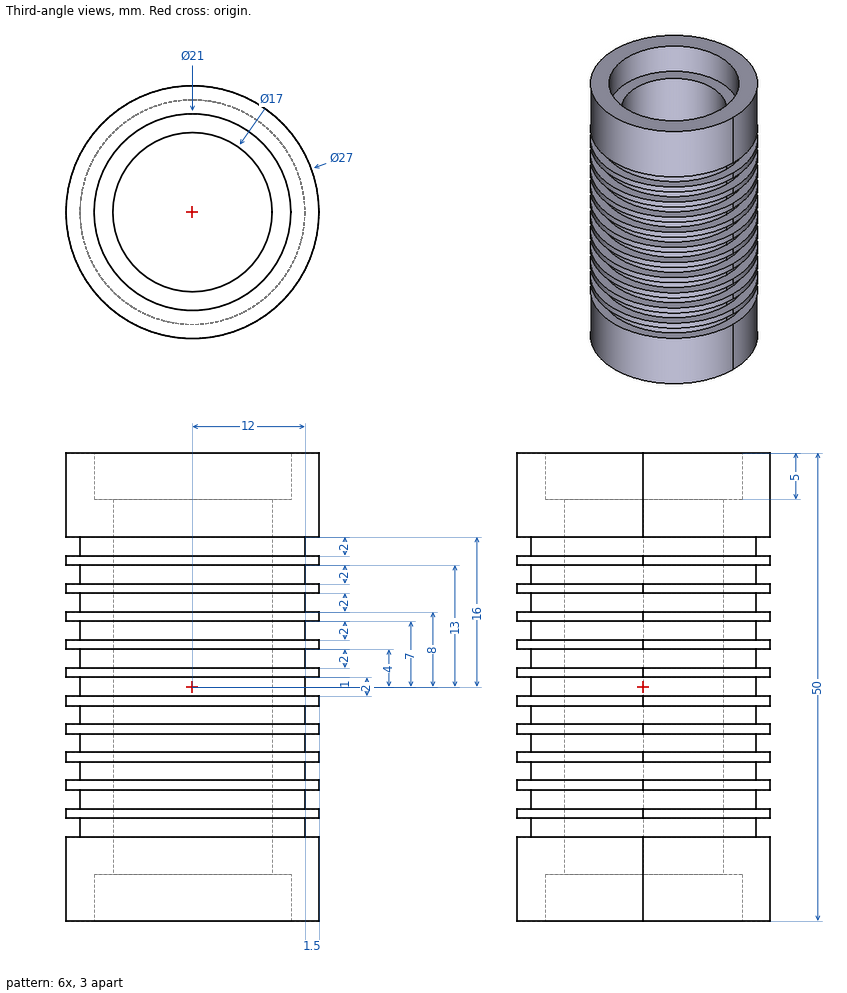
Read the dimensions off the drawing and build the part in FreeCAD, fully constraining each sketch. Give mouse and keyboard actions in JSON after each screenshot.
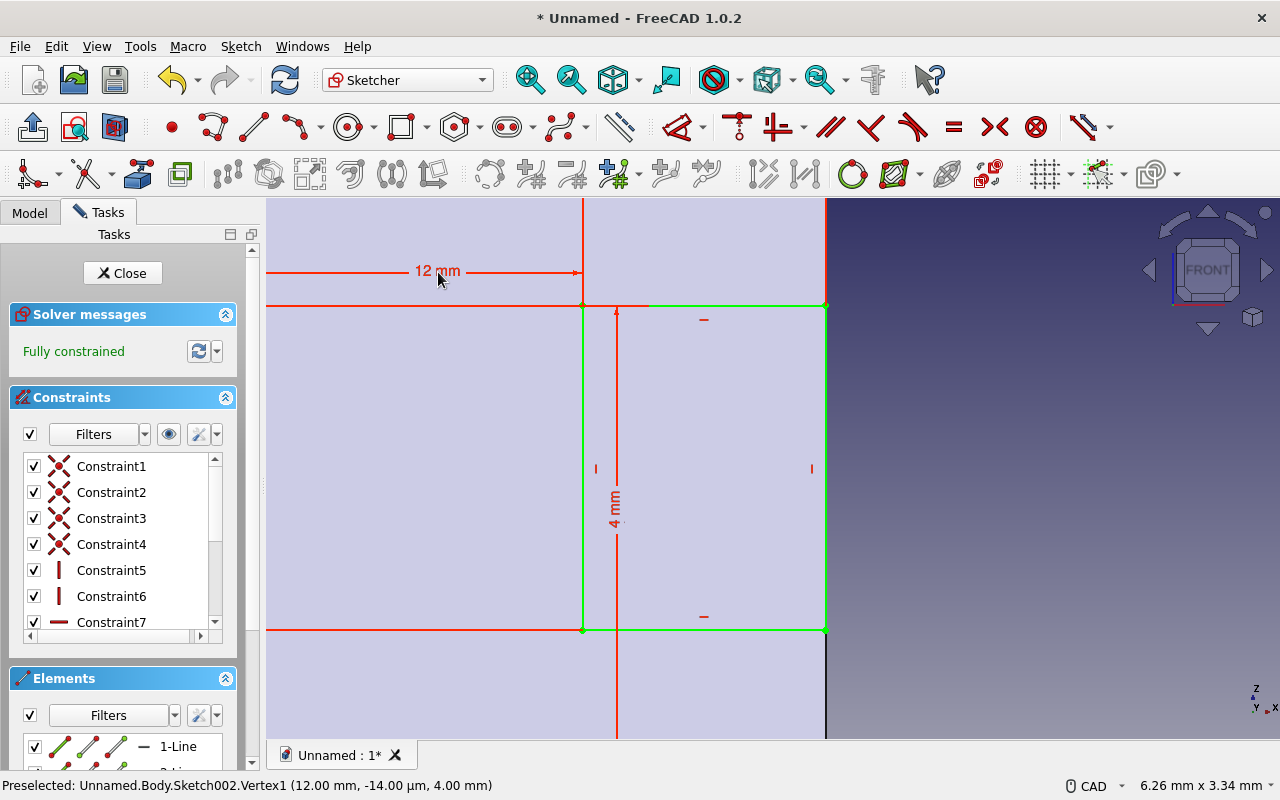
{"action": "left_click", "coordinate": [123, 273]}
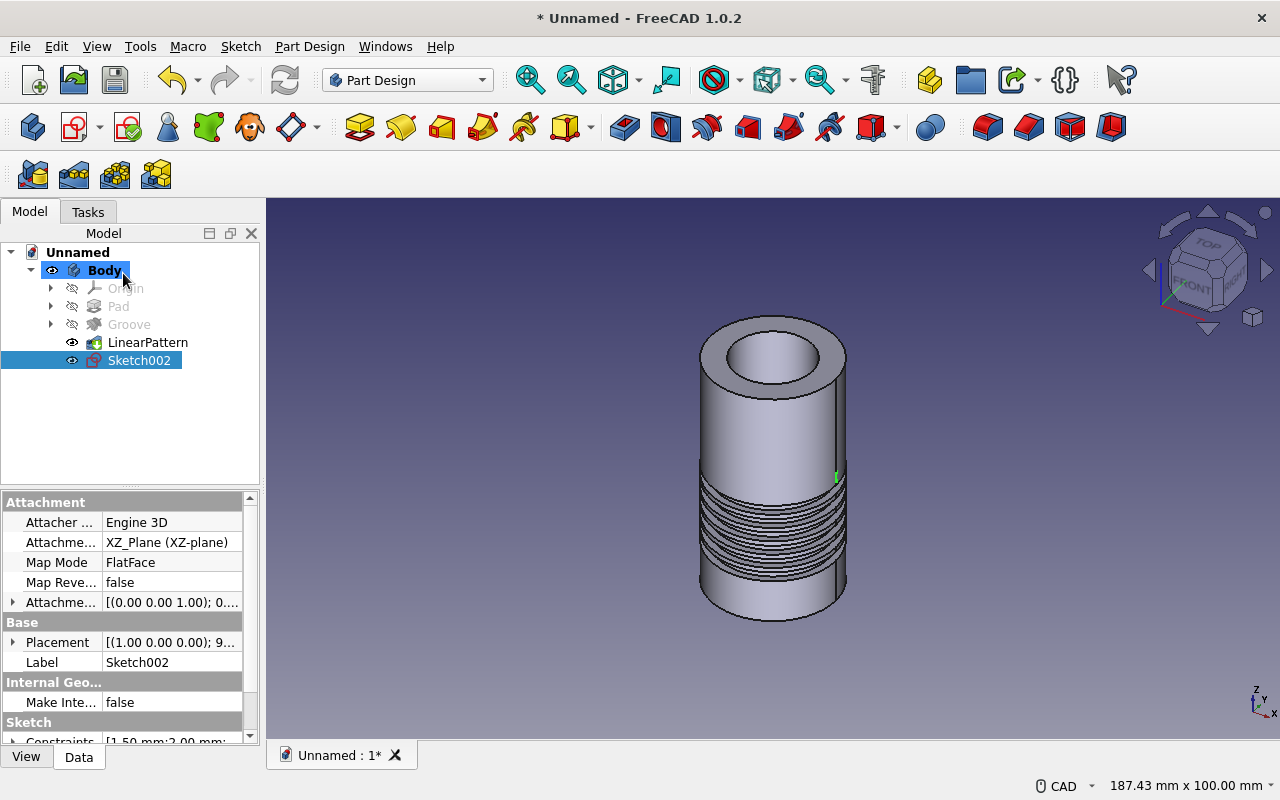
{"action": "left_click", "coordinate": [707, 128]}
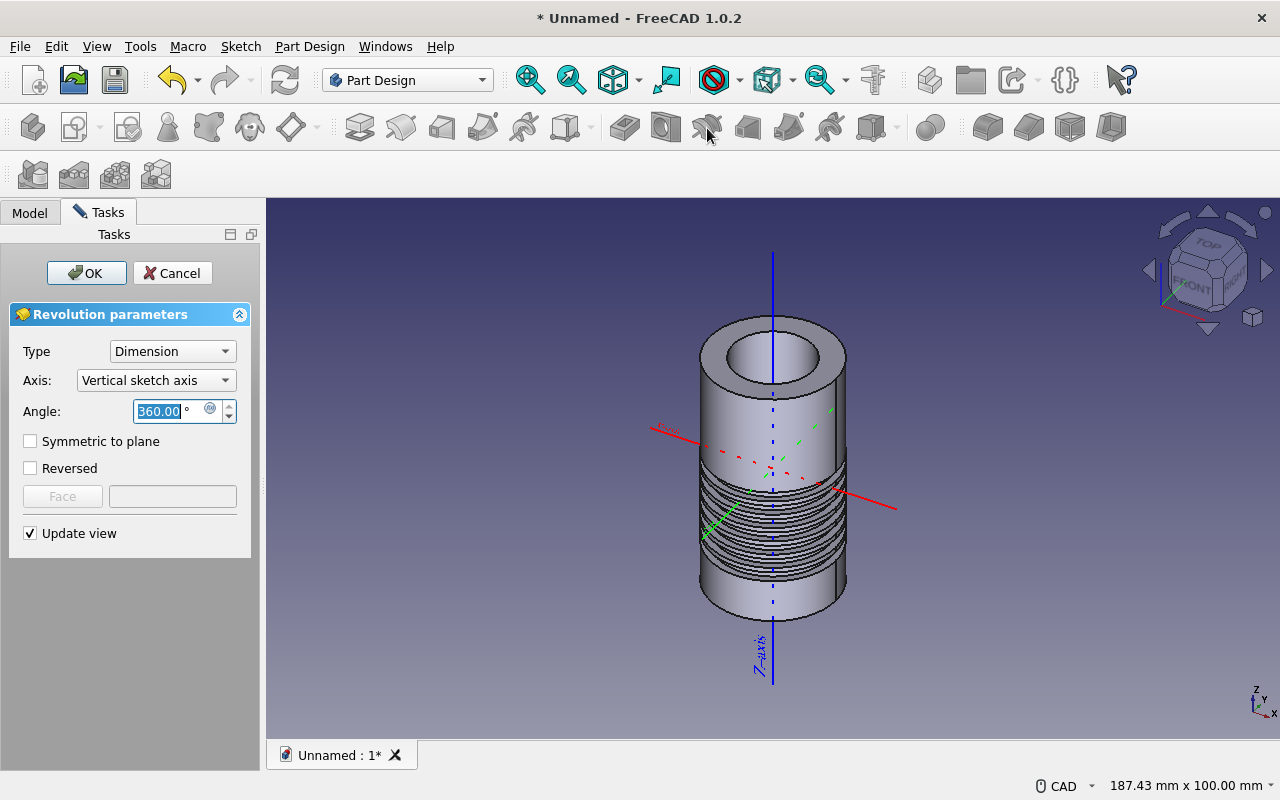
{"action": "left_click", "coordinate": [87, 273]}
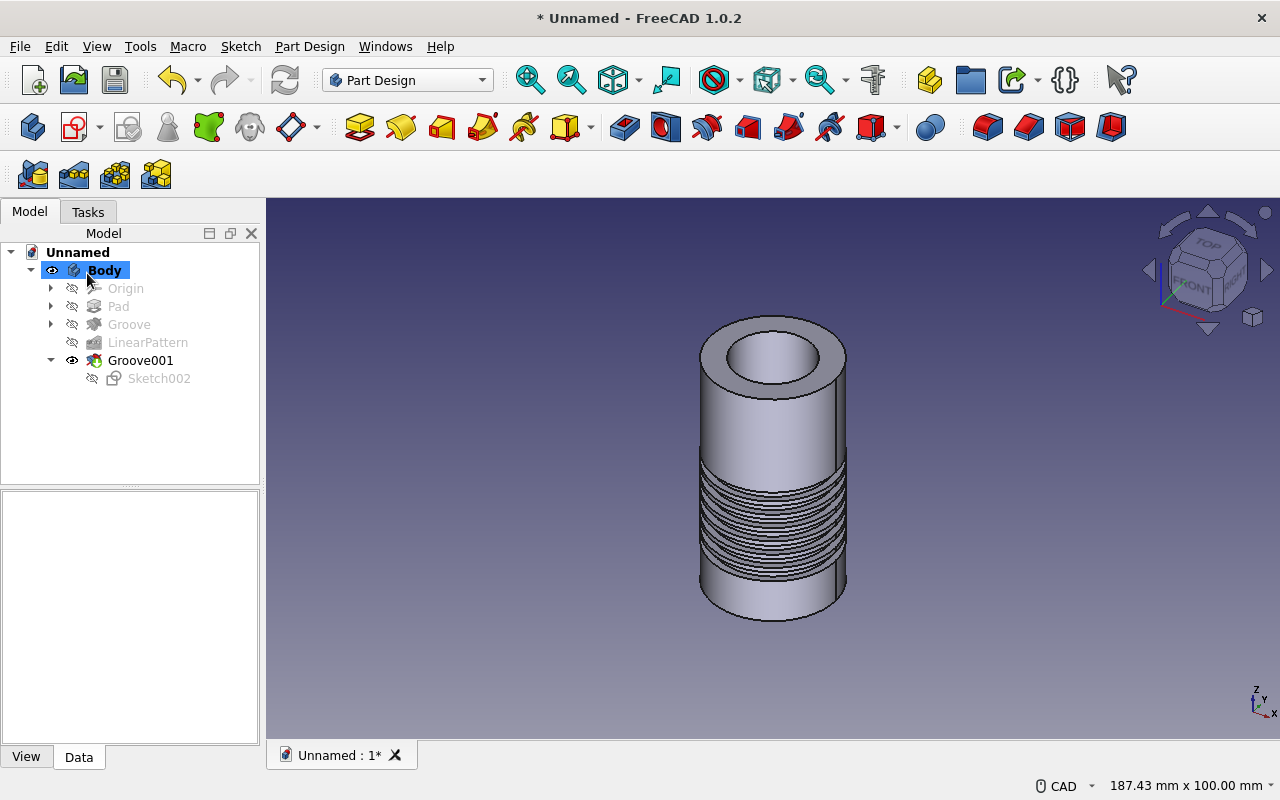
{"action": "left_click", "coordinate": [74, 128]}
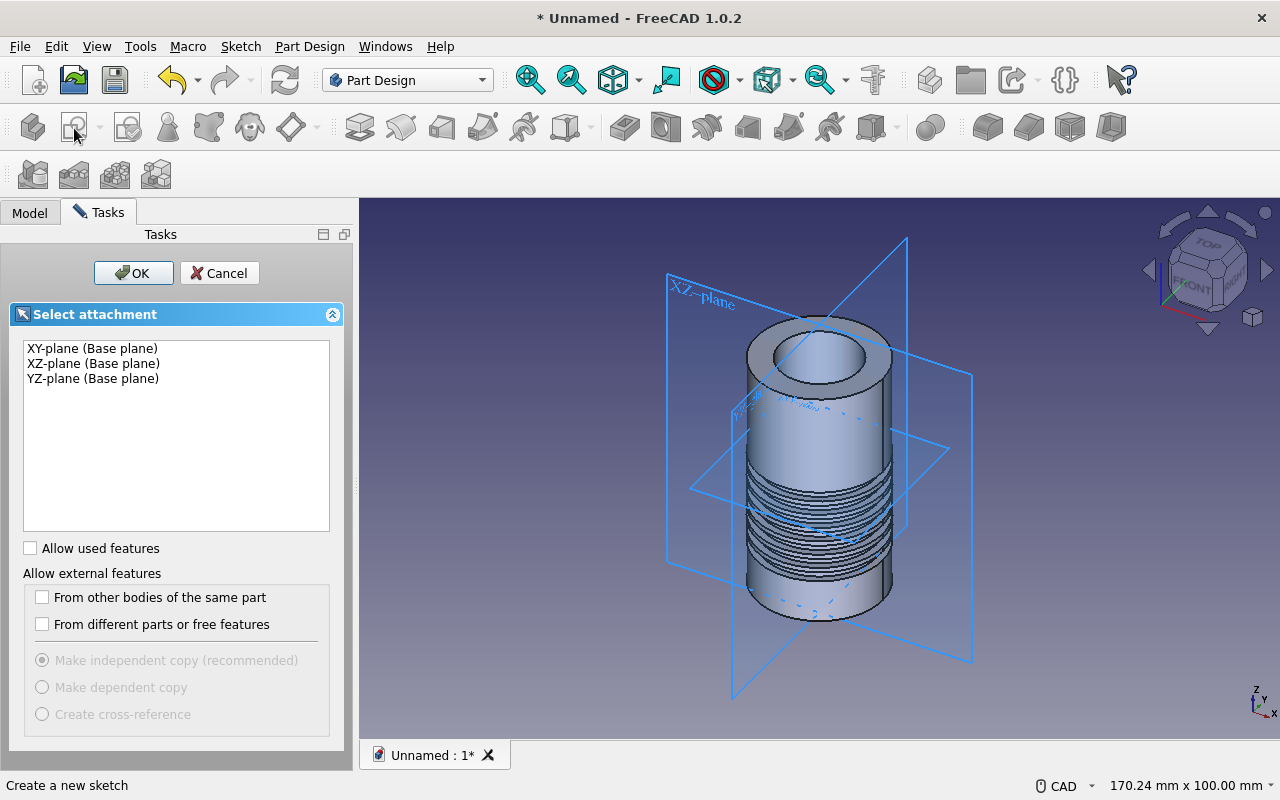
{"action": "left_click", "coordinate": [84, 364]}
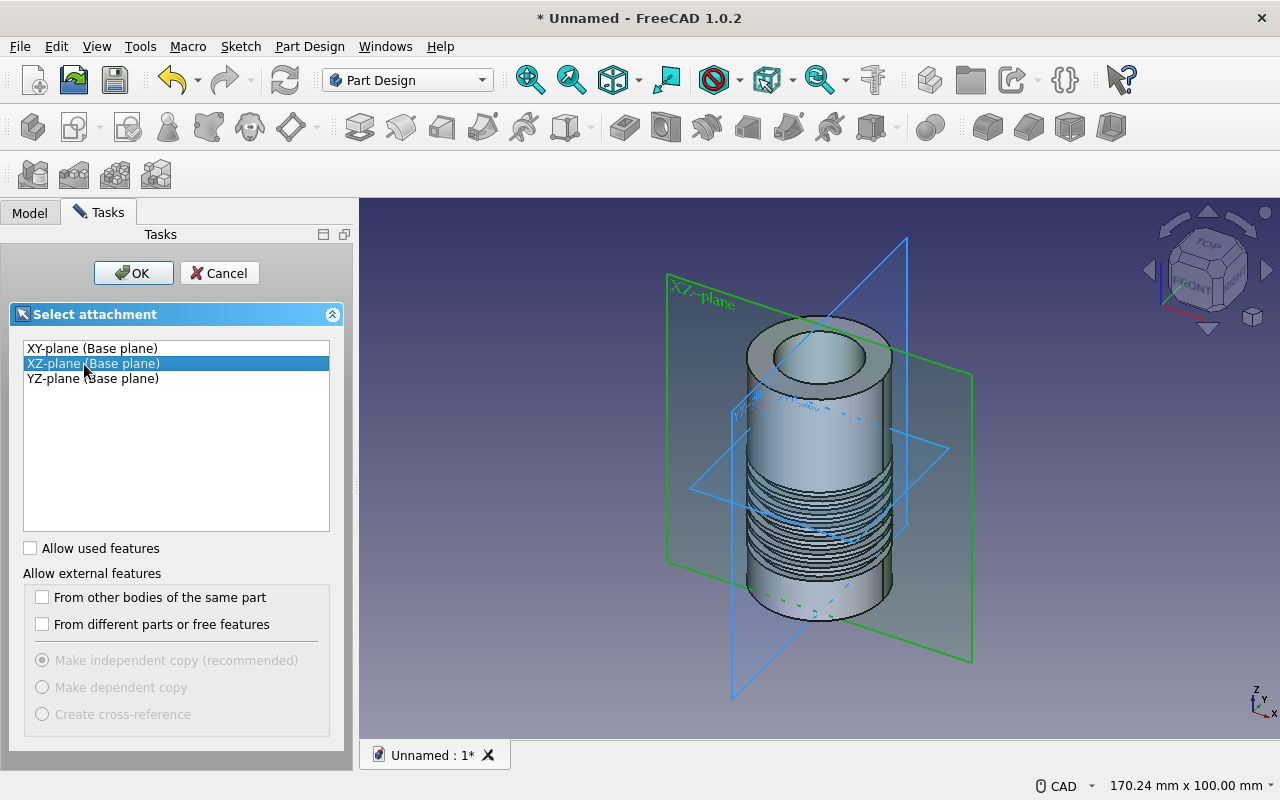
{"action": "left_click", "coordinate": [134, 273]}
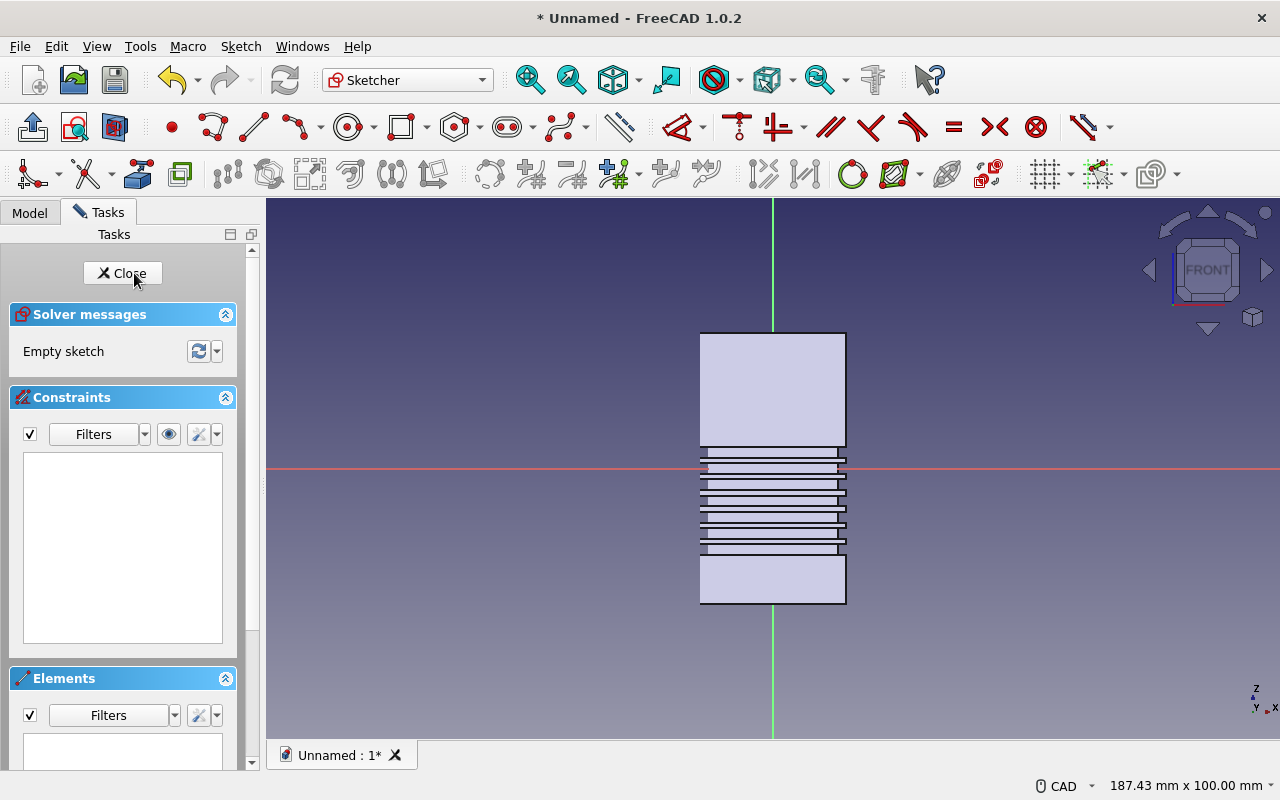
{"action": "left_click", "coordinate": [115, 128]}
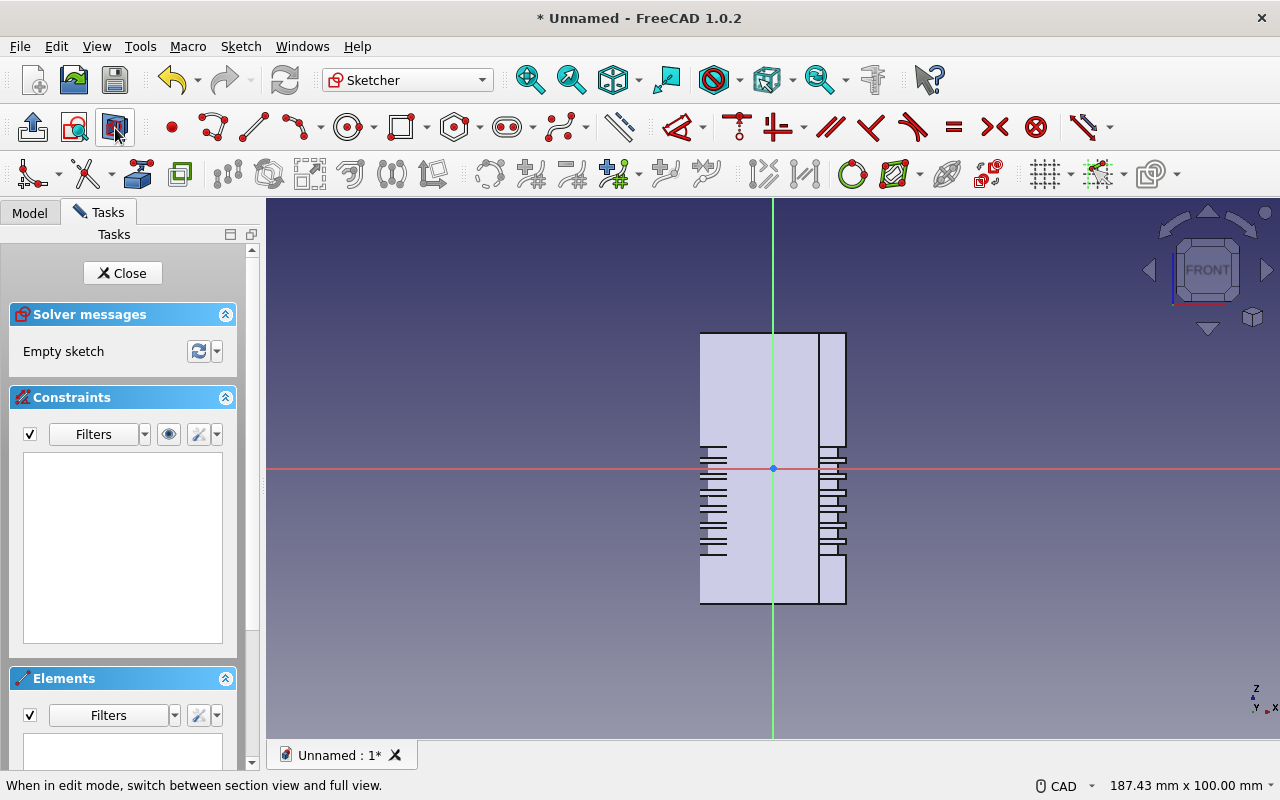
{"action": "scroll", "coordinate": [849, 434], "scroll_direction": "up", "scroll_amount": 15}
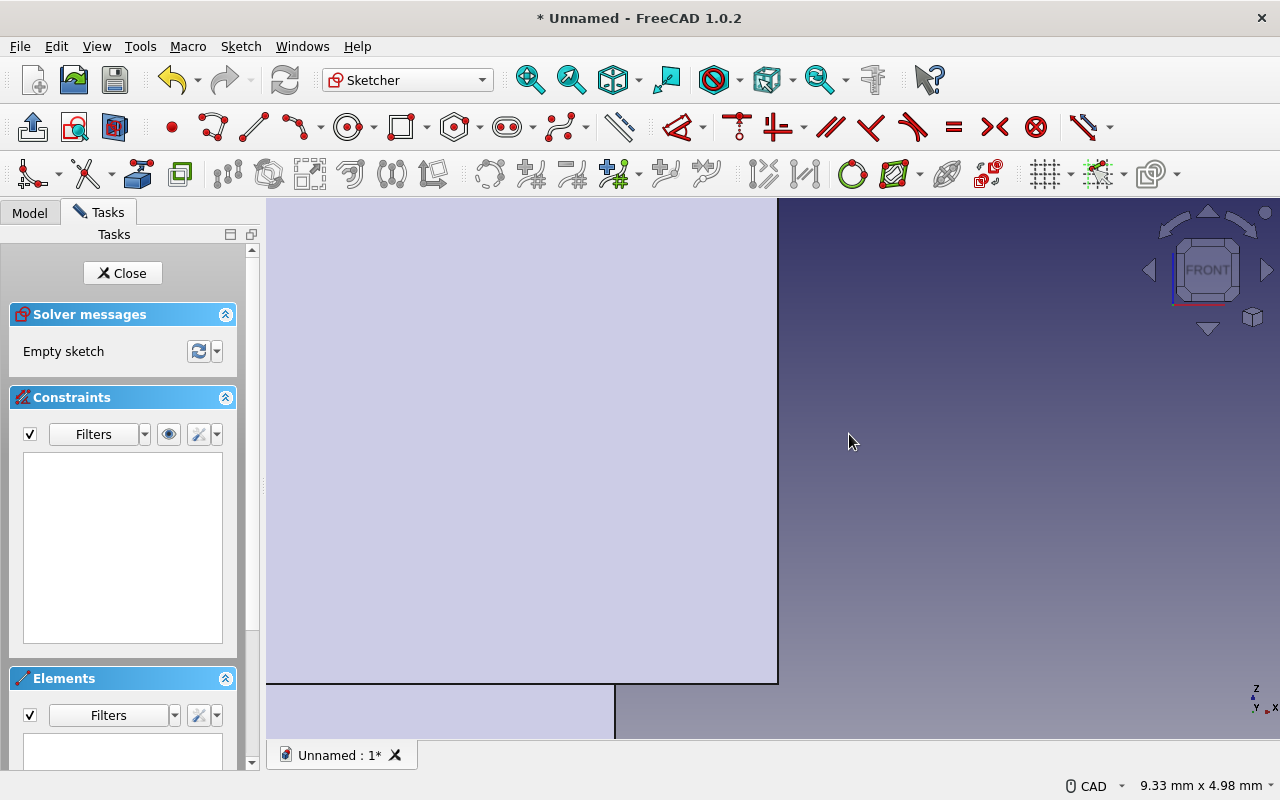
{"action": "scroll", "coordinate": [682, 463], "scroll_direction": "up", "scroll_amount": 2}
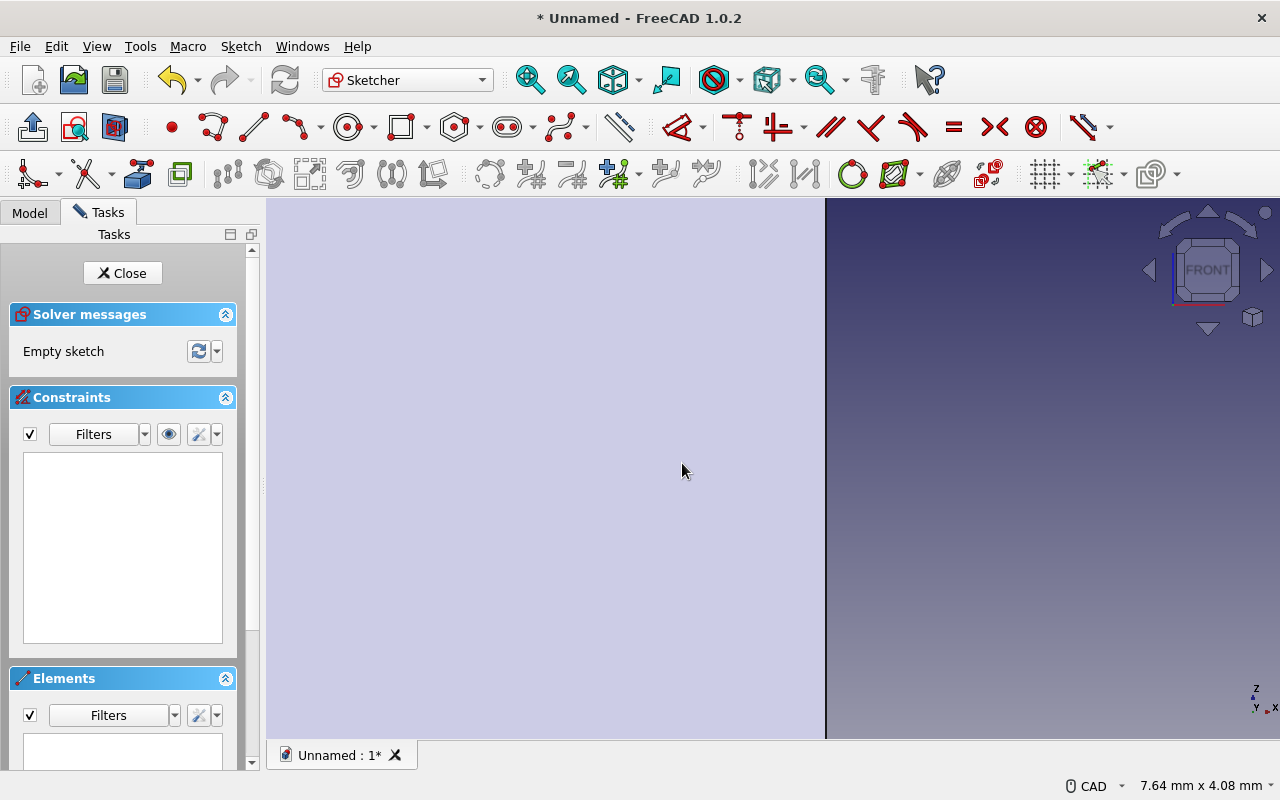
{"action": "left_click", "coordinate": [400, 128]}